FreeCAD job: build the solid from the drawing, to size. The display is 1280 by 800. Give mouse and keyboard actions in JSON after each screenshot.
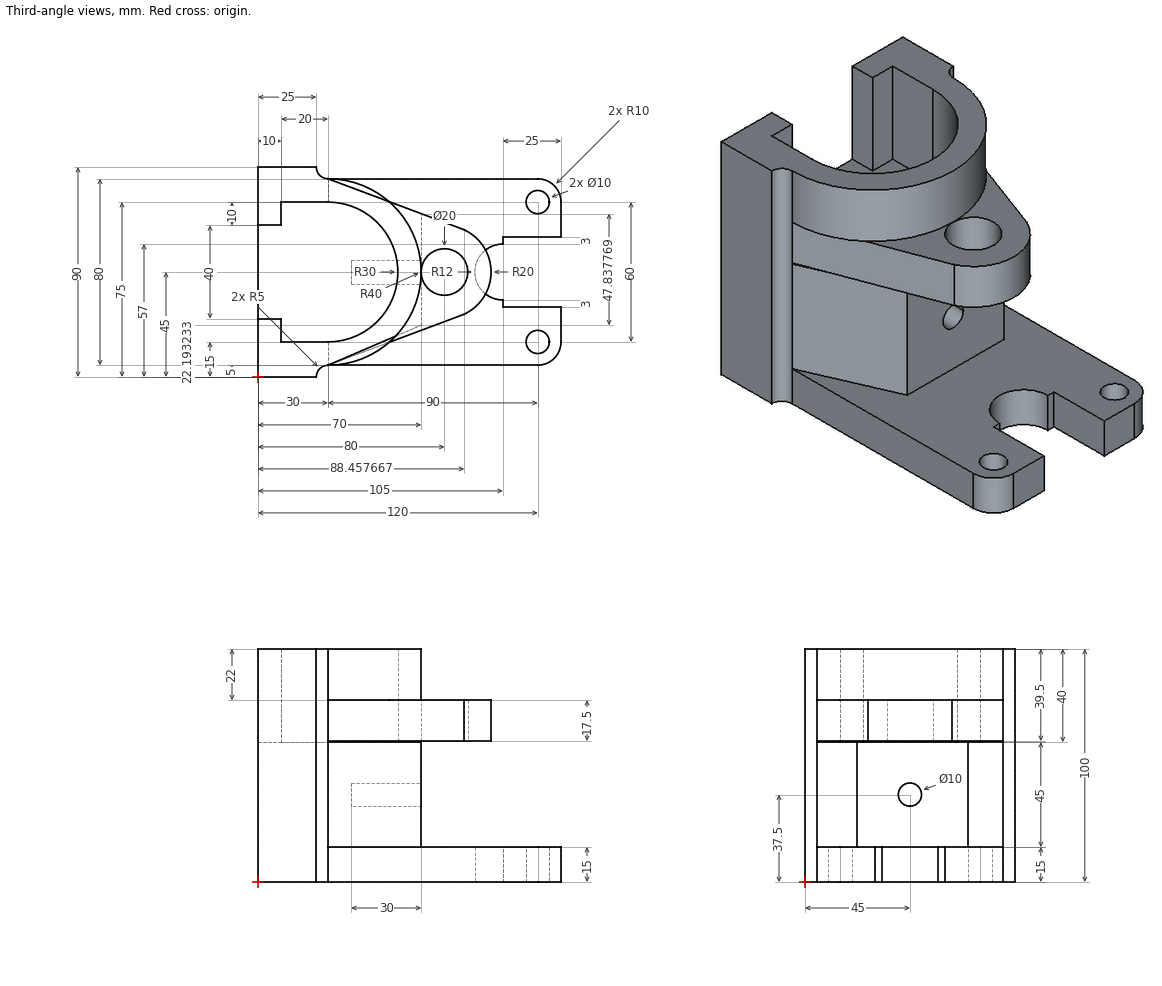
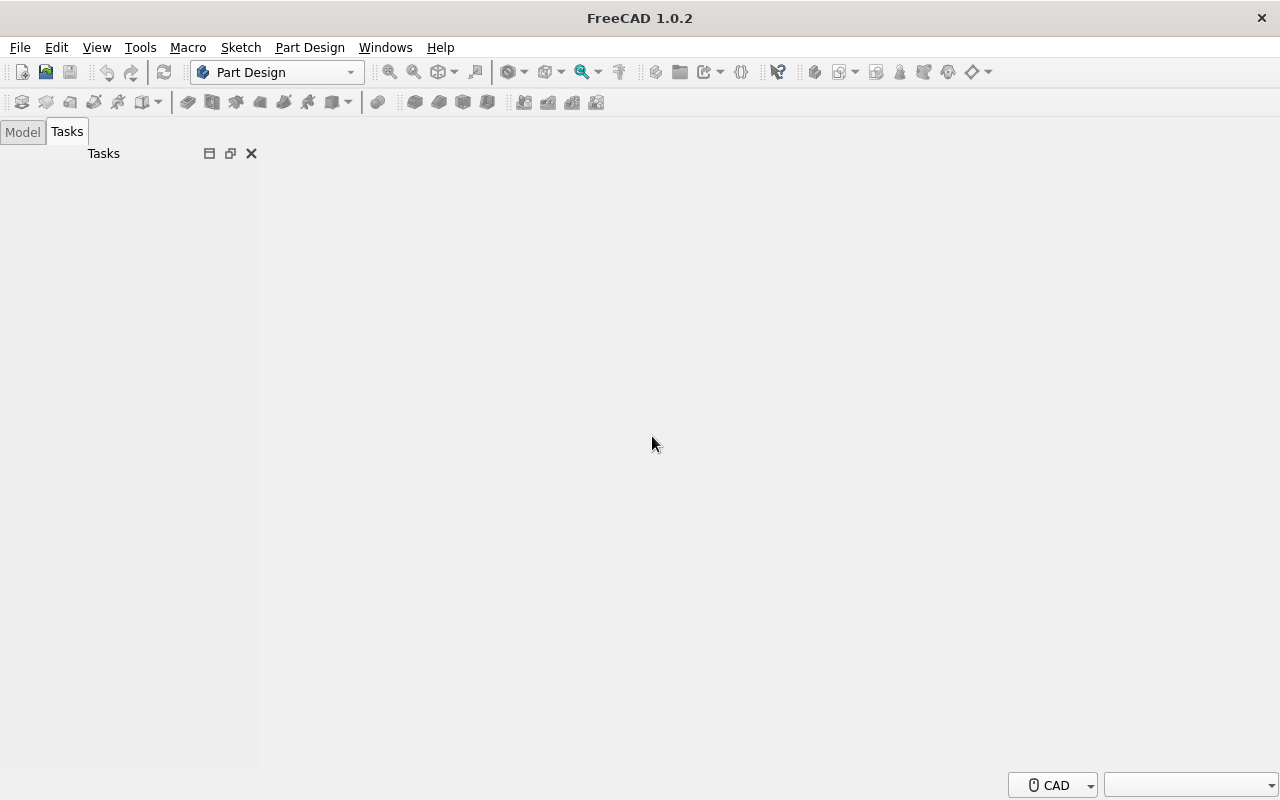
{"action": "left_click", "coordinate": [22, 72]}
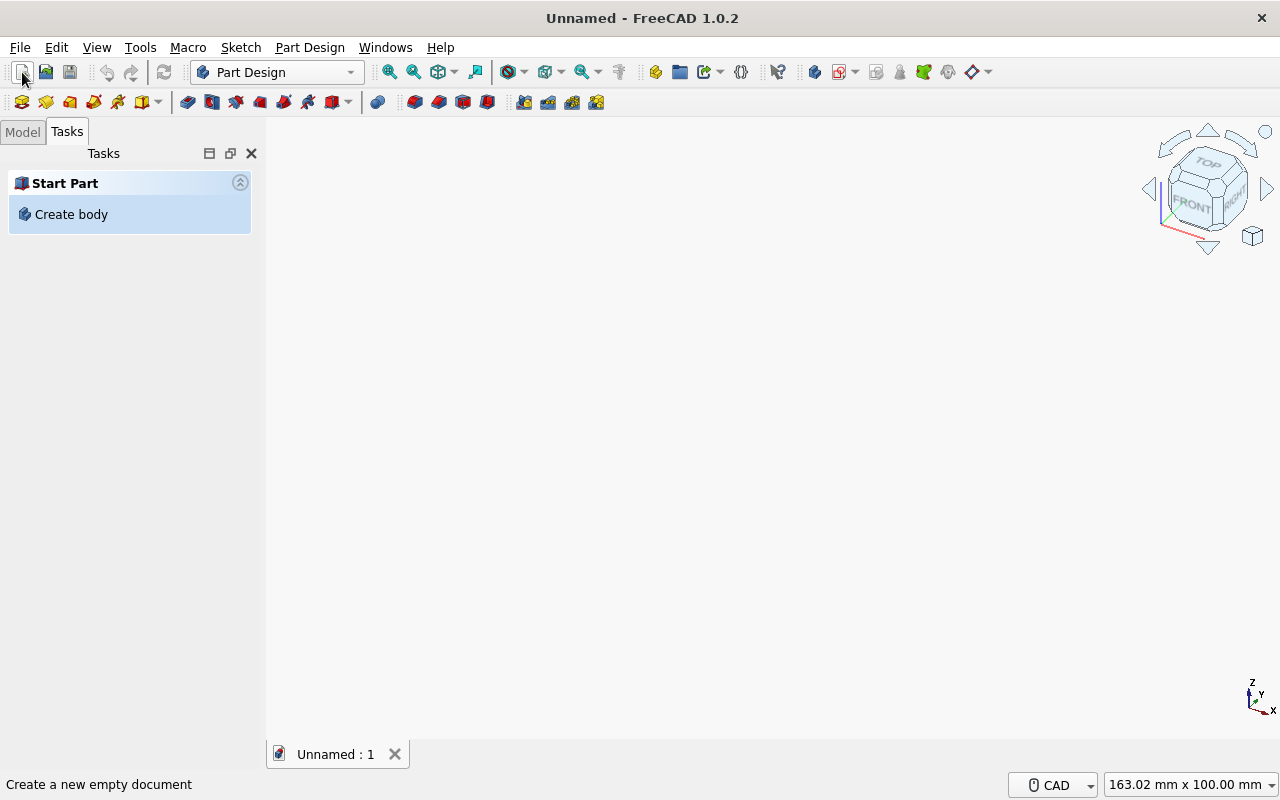
{"action": "left_click", "coordinate": [840, 72]}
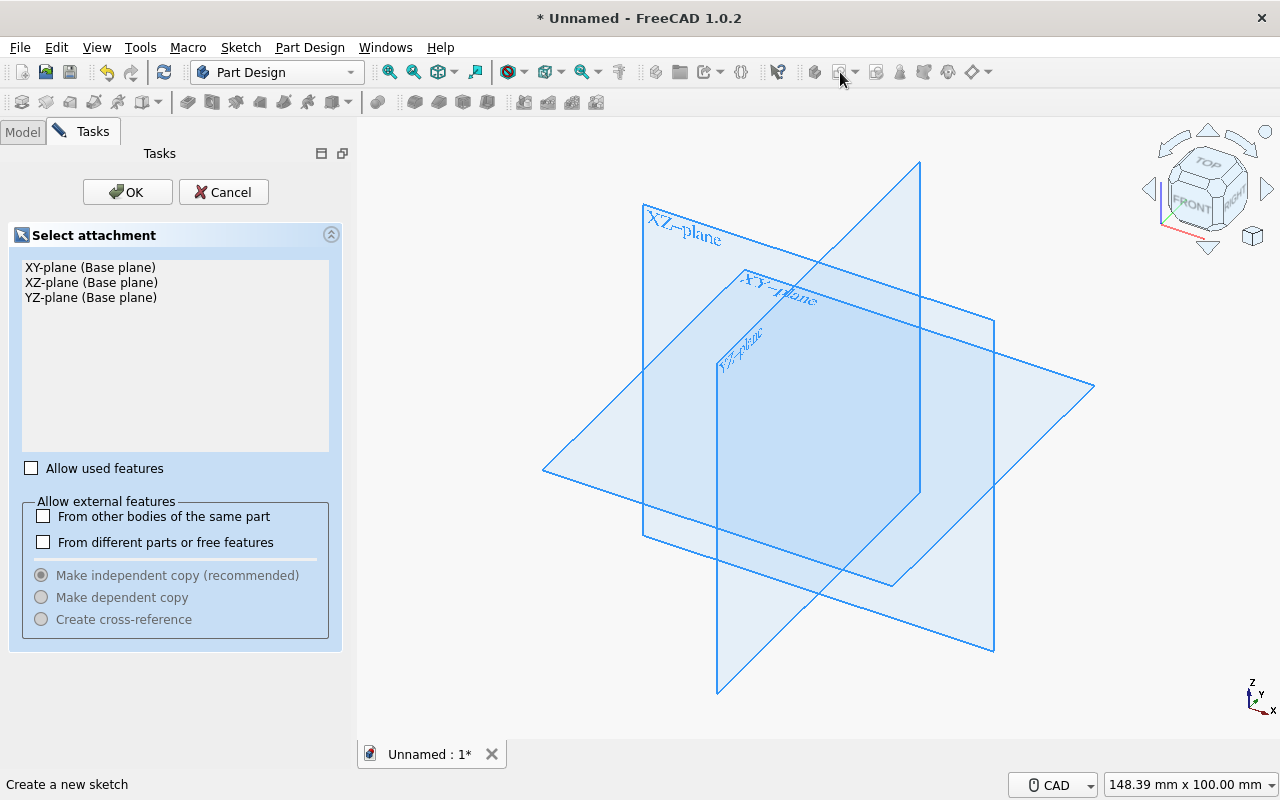
{"action": "left_click", "coordinate": [82, 268]}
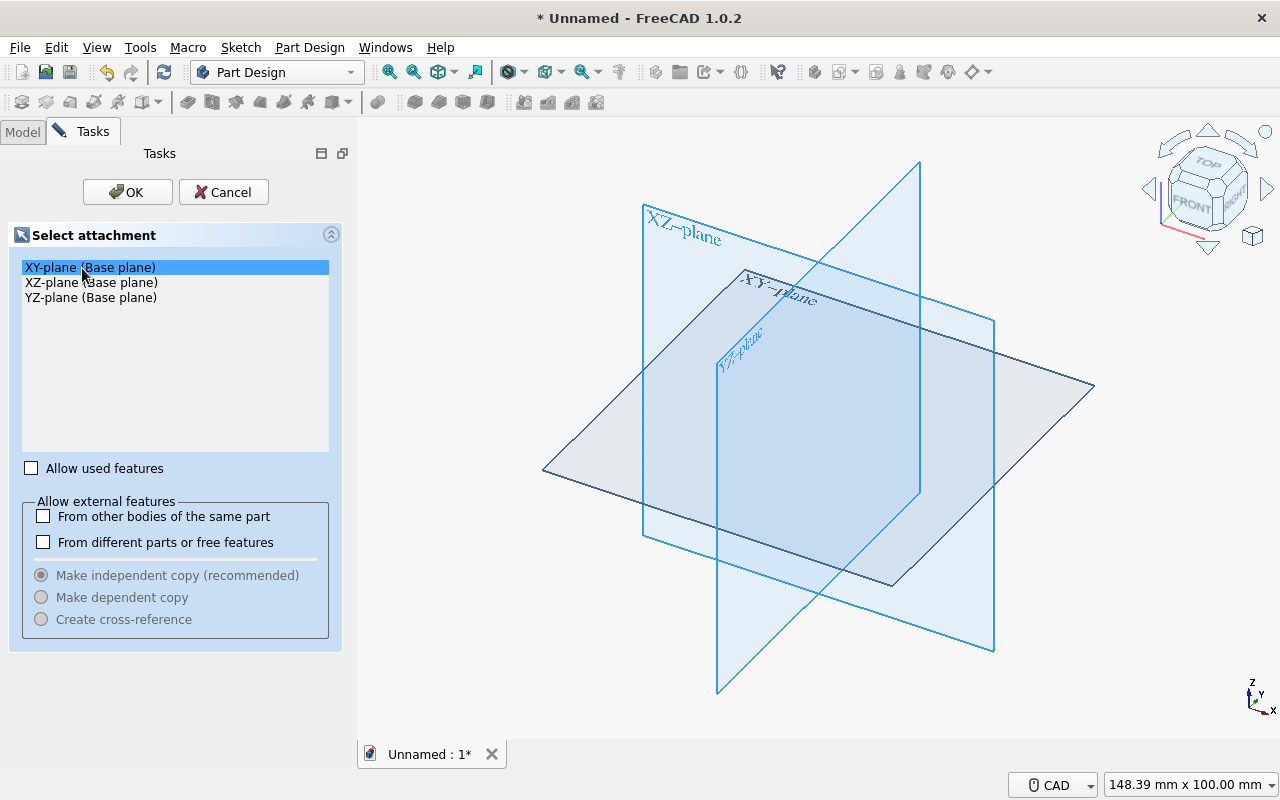
{"action": "left_click", "coordinate": [128, 192]}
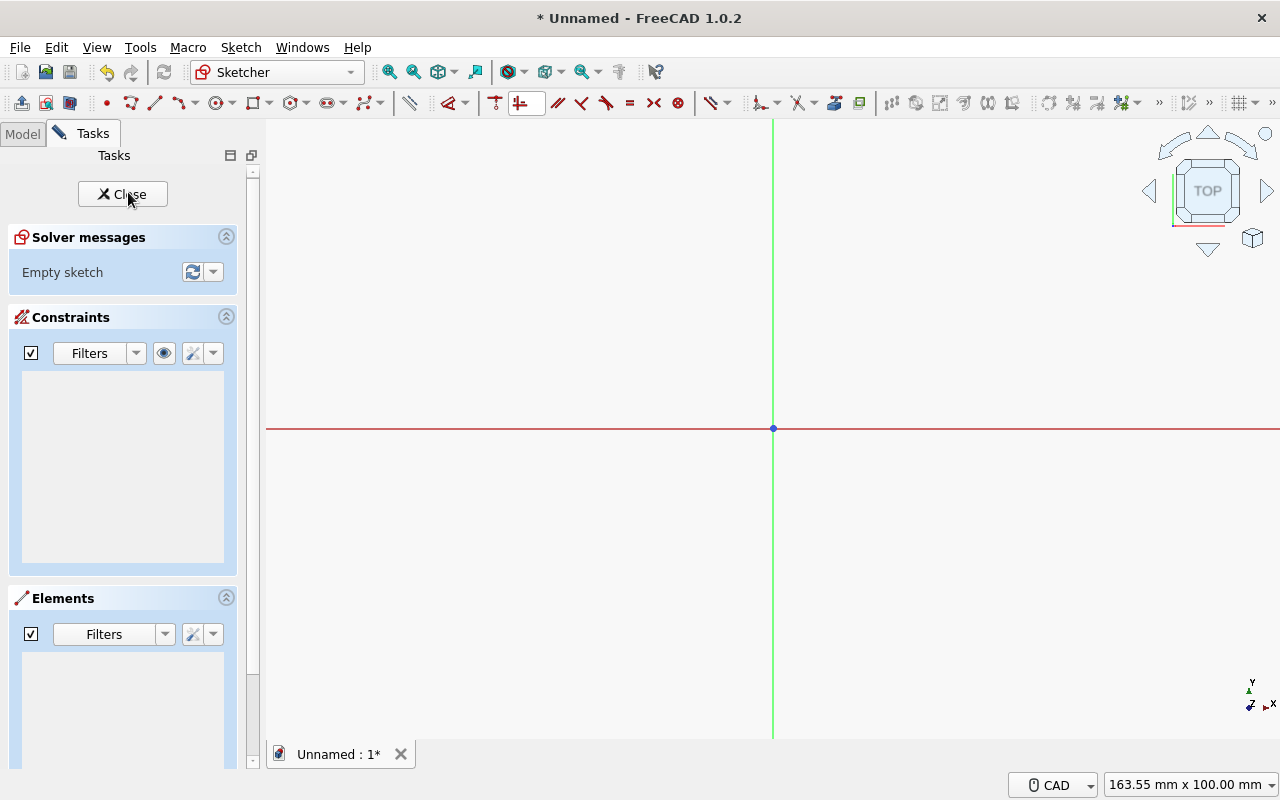
{"action": "scroll", "coordinate": [508, 711], "scroll_direction": "down", "scroll_amount": 3}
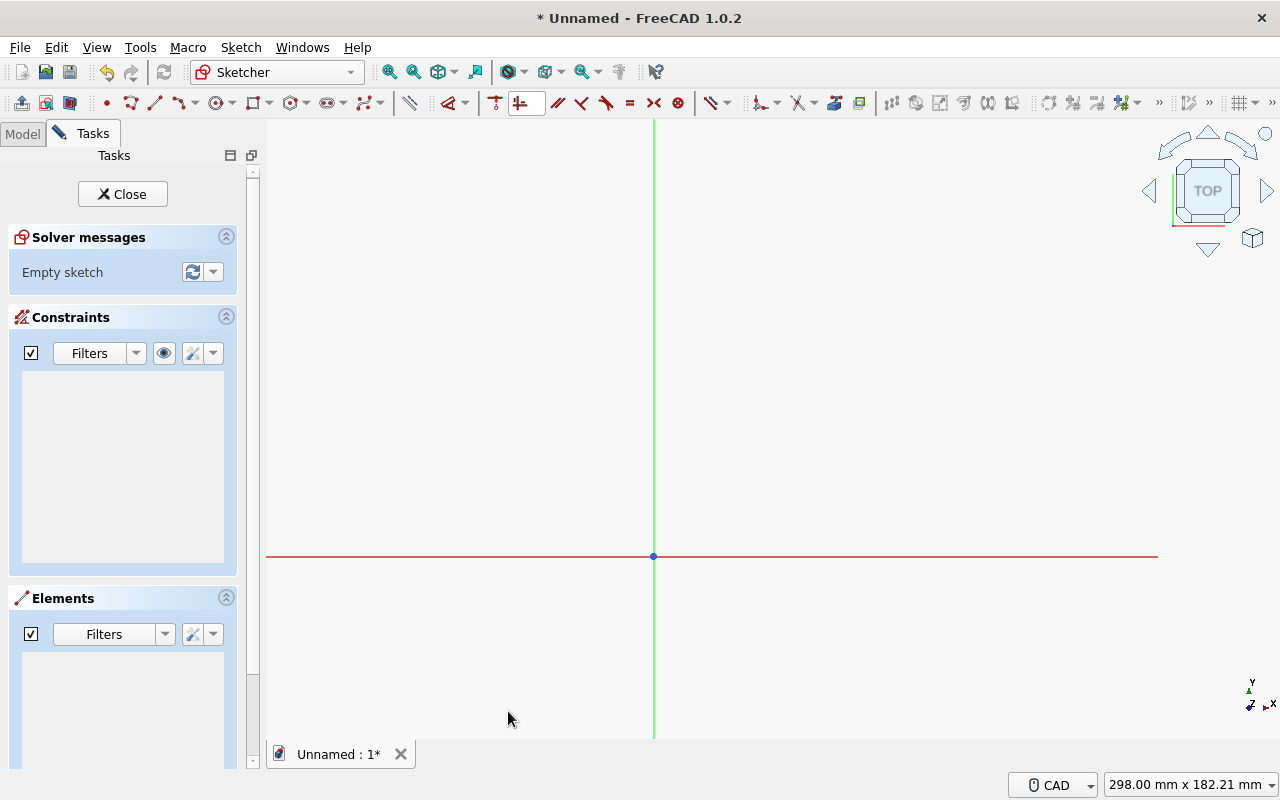
{"action": "left_click", "coordinate": [156, 104]}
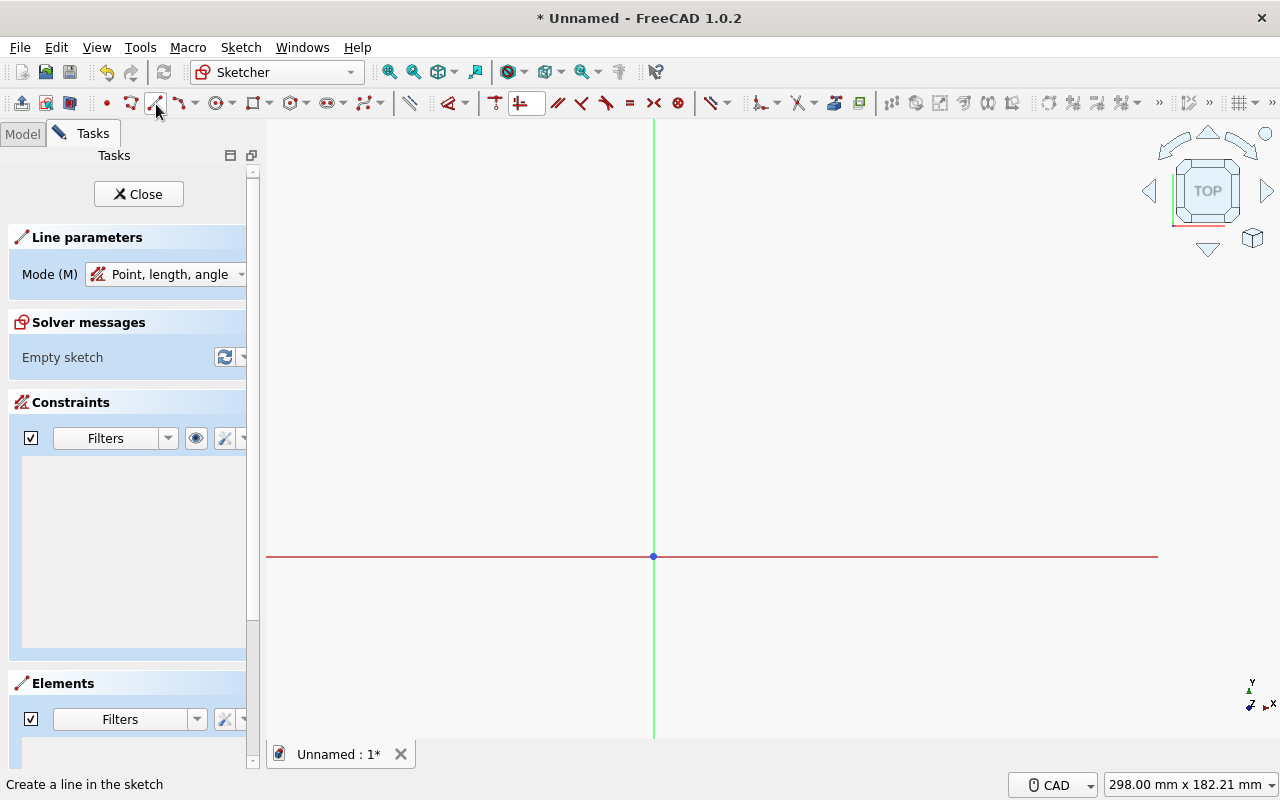
{"action": "left_click", "coordinate": [756, 540]}
{"action": "left_click", "coordinate": [756, 267]}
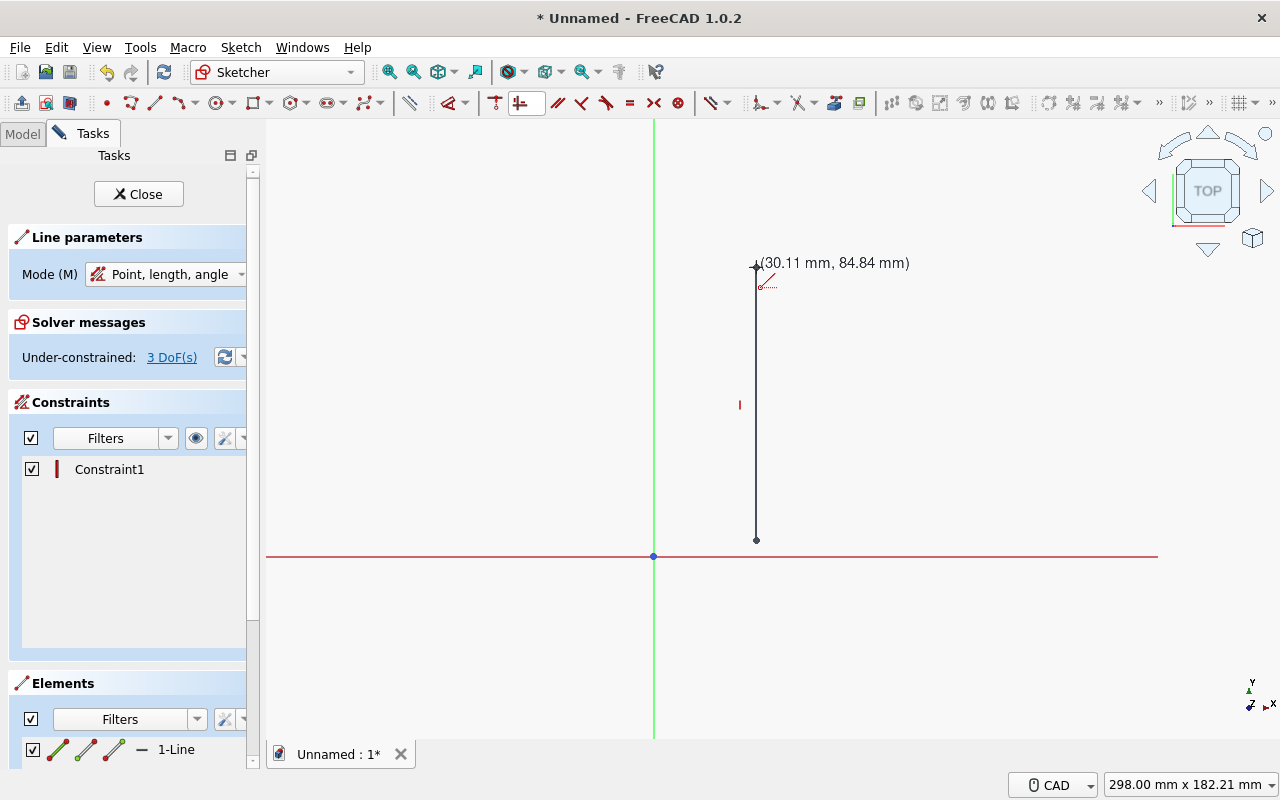
{"action": "left_click", "coordinate": [132, 104]}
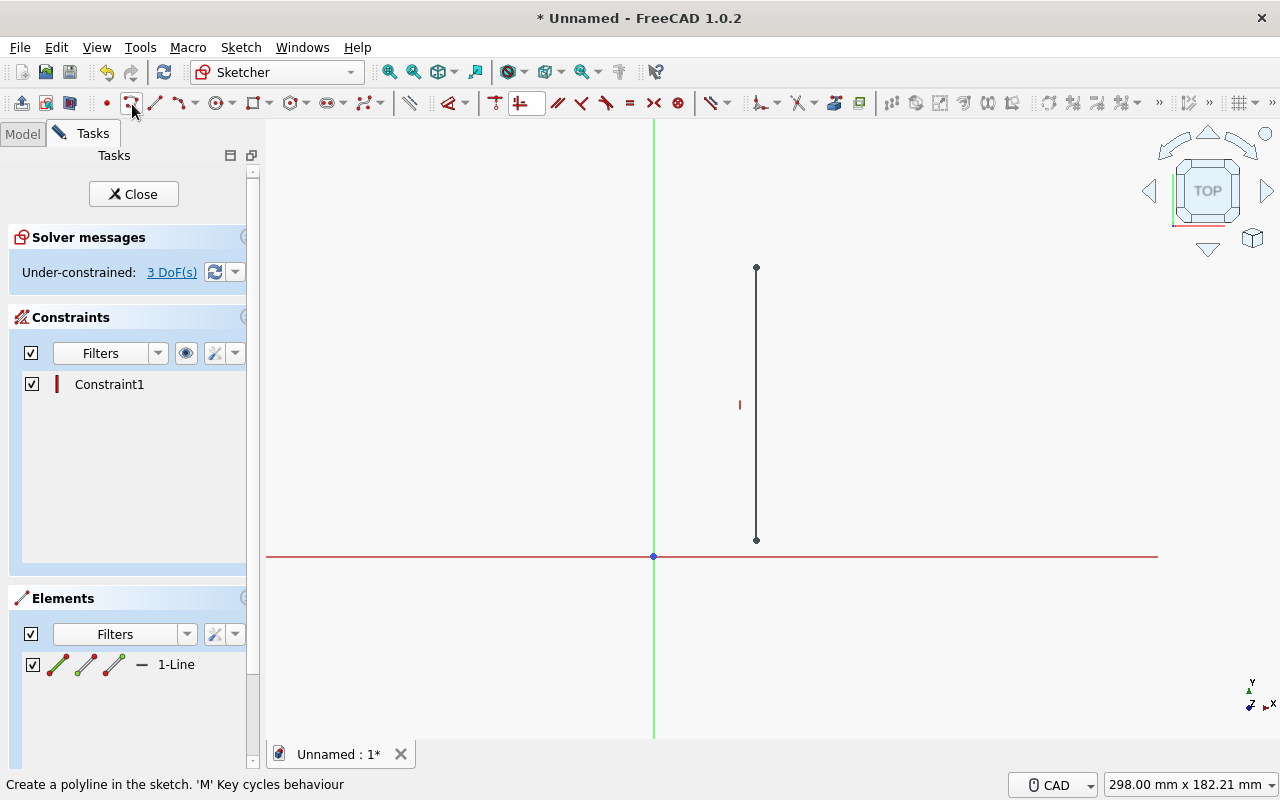
{"action": "left_click", "coordinate": [739, 250]}
{"action": "left_click", "coordinate": [654, 250]}
{"action": "left_click", "coordinate": [654, 557]}
{"action": "left_click", "coordinate": [739, 548]}
{"action": "right_click", "coordinate": [739, 548]}